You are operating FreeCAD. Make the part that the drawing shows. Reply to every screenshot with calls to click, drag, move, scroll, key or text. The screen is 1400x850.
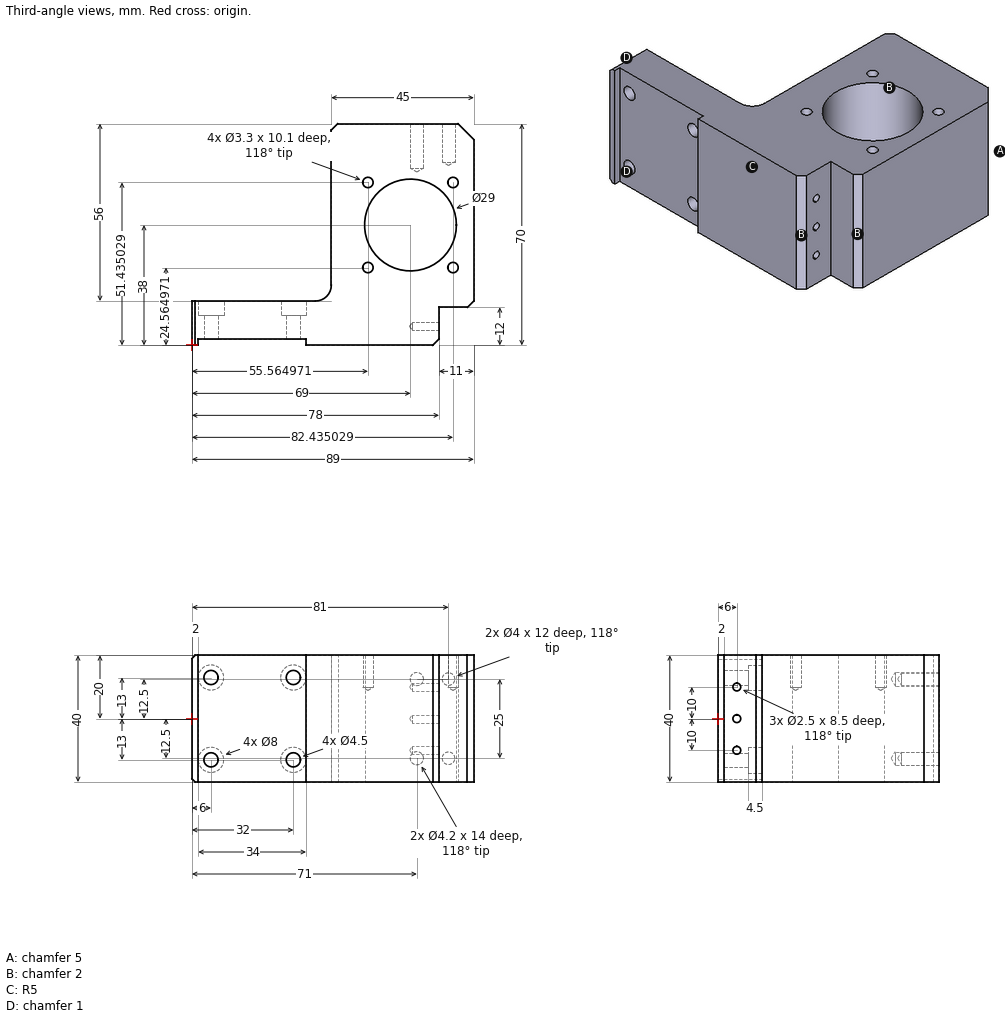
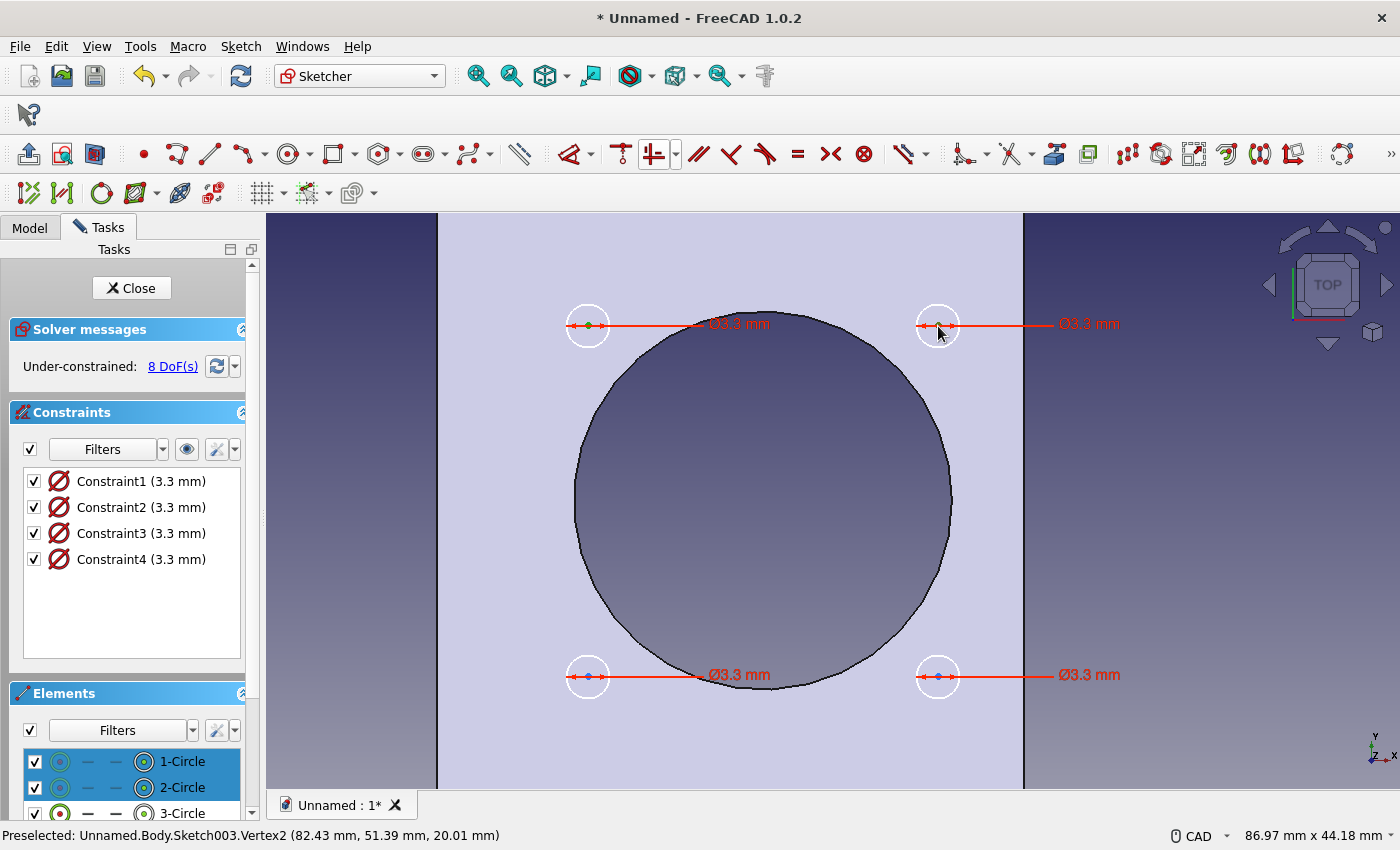
click(676, 154)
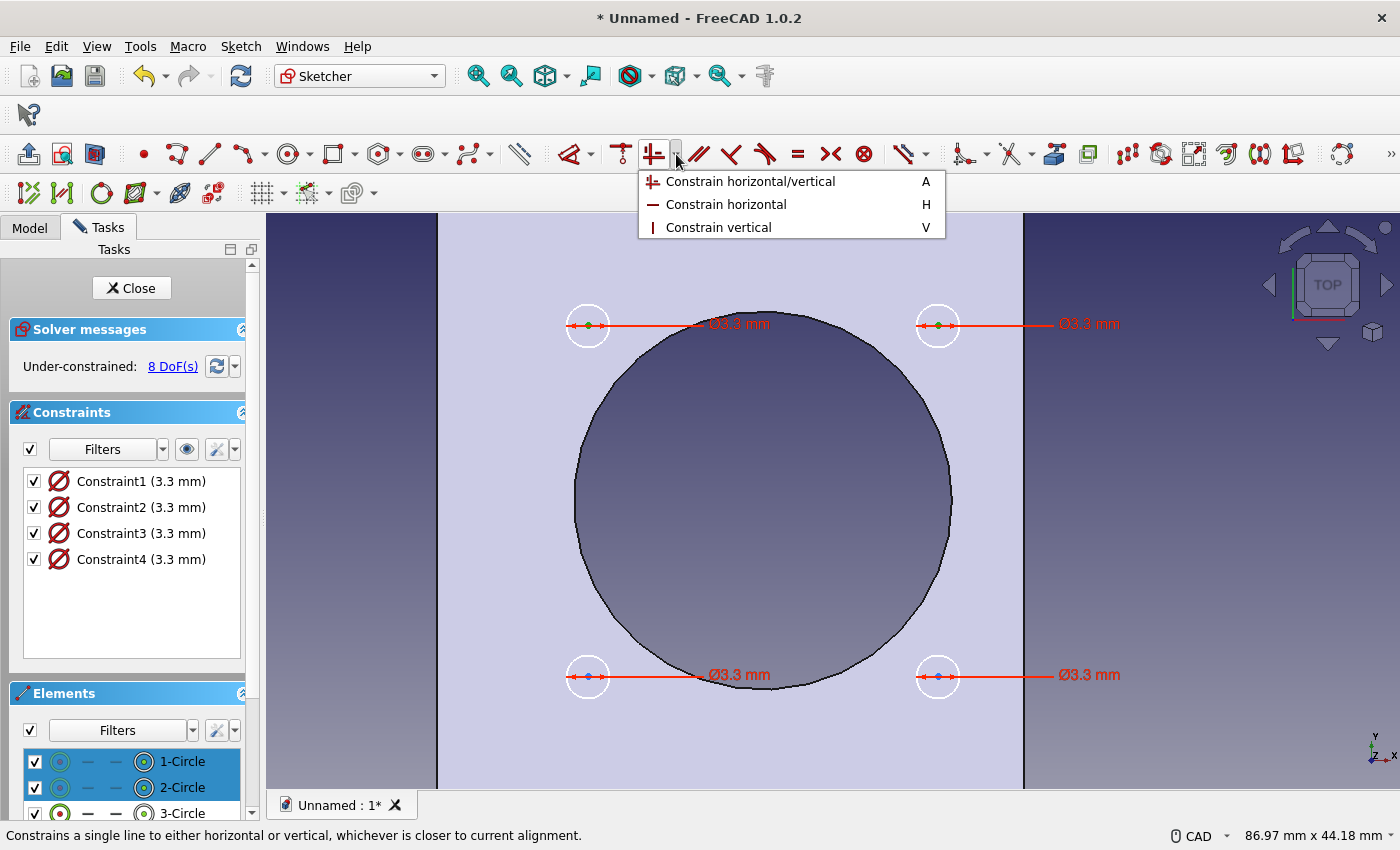
click(792, 204)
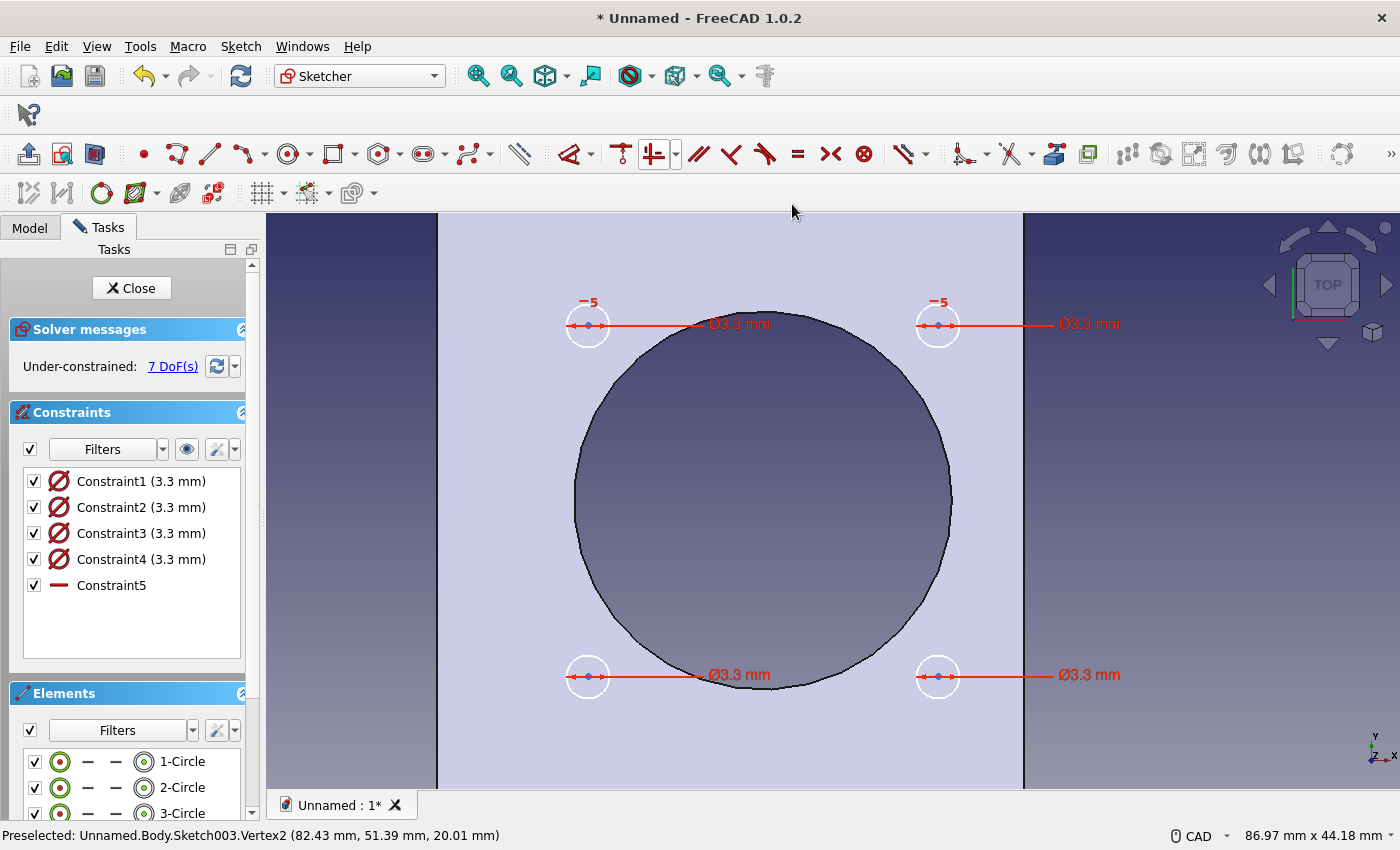
click(588, 326)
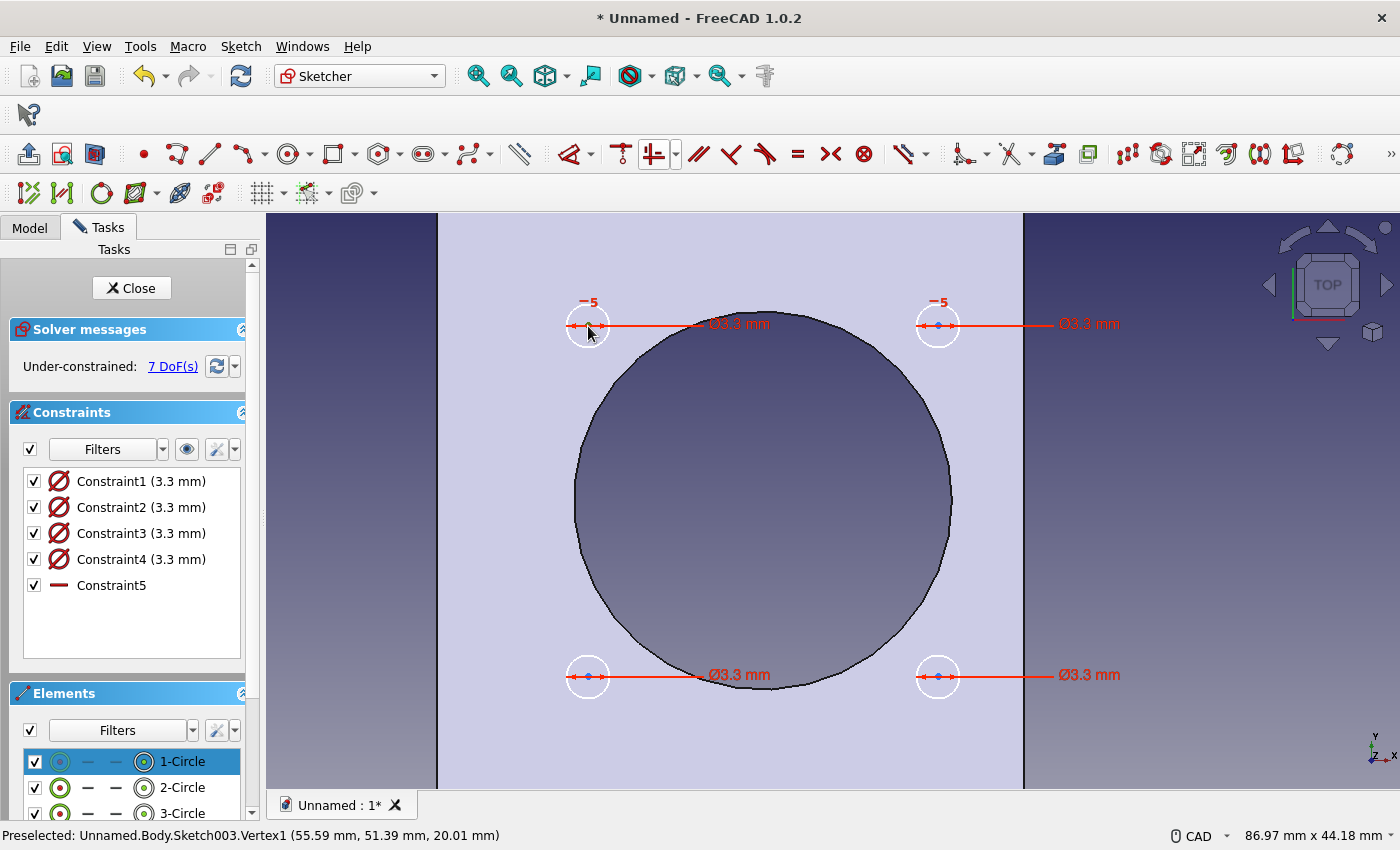
click(588, 677)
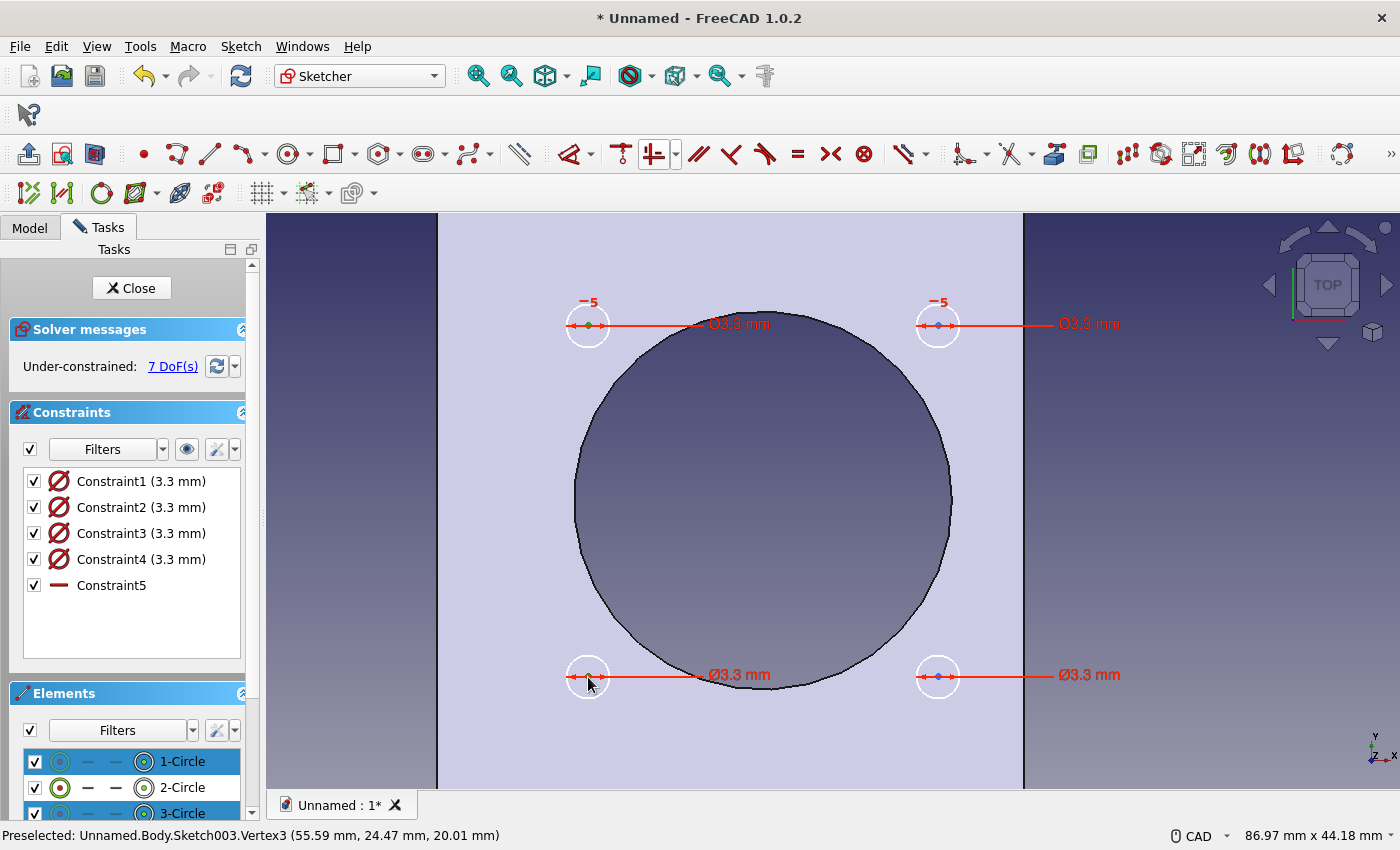
click(676, 154)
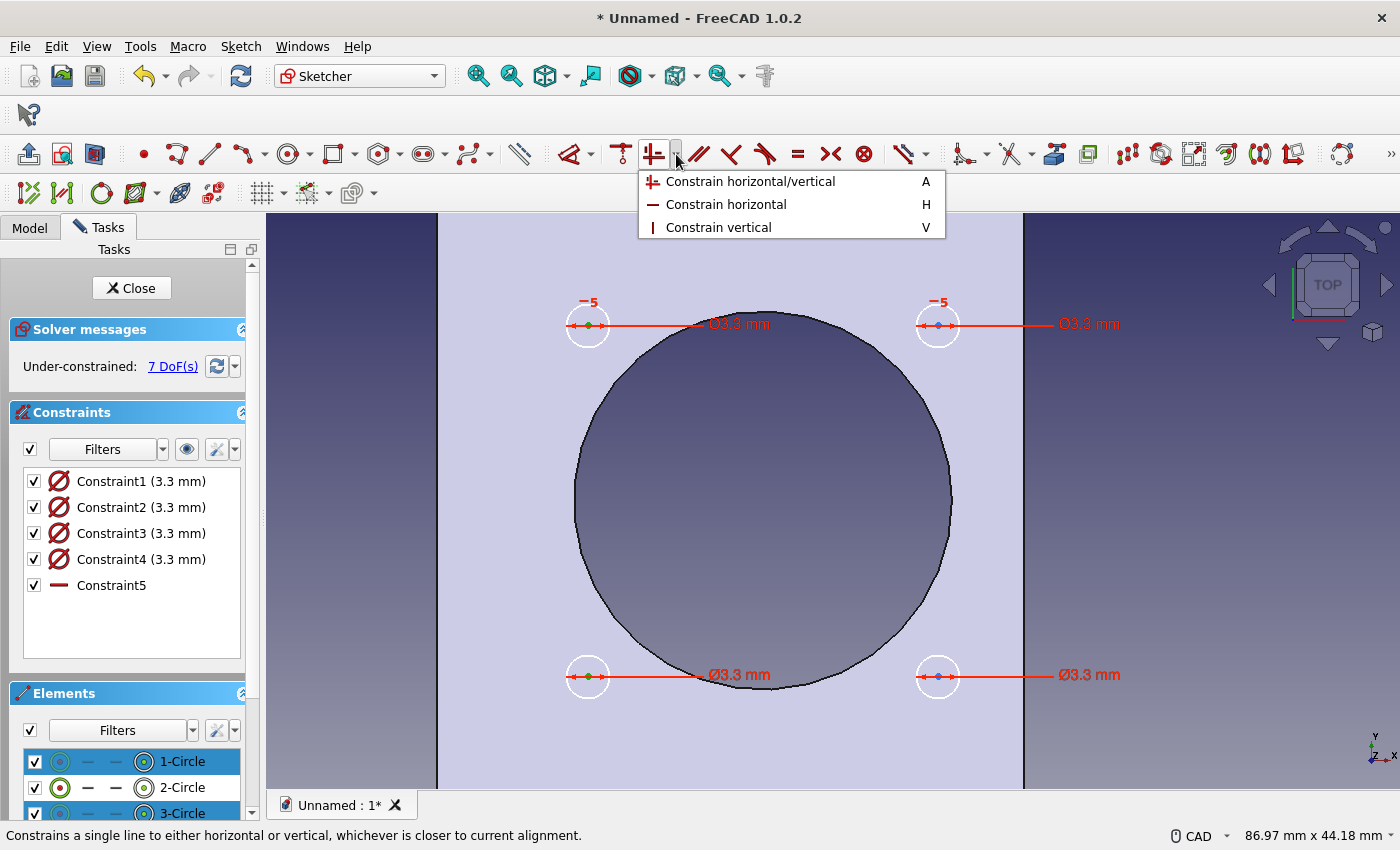
click(792, 228)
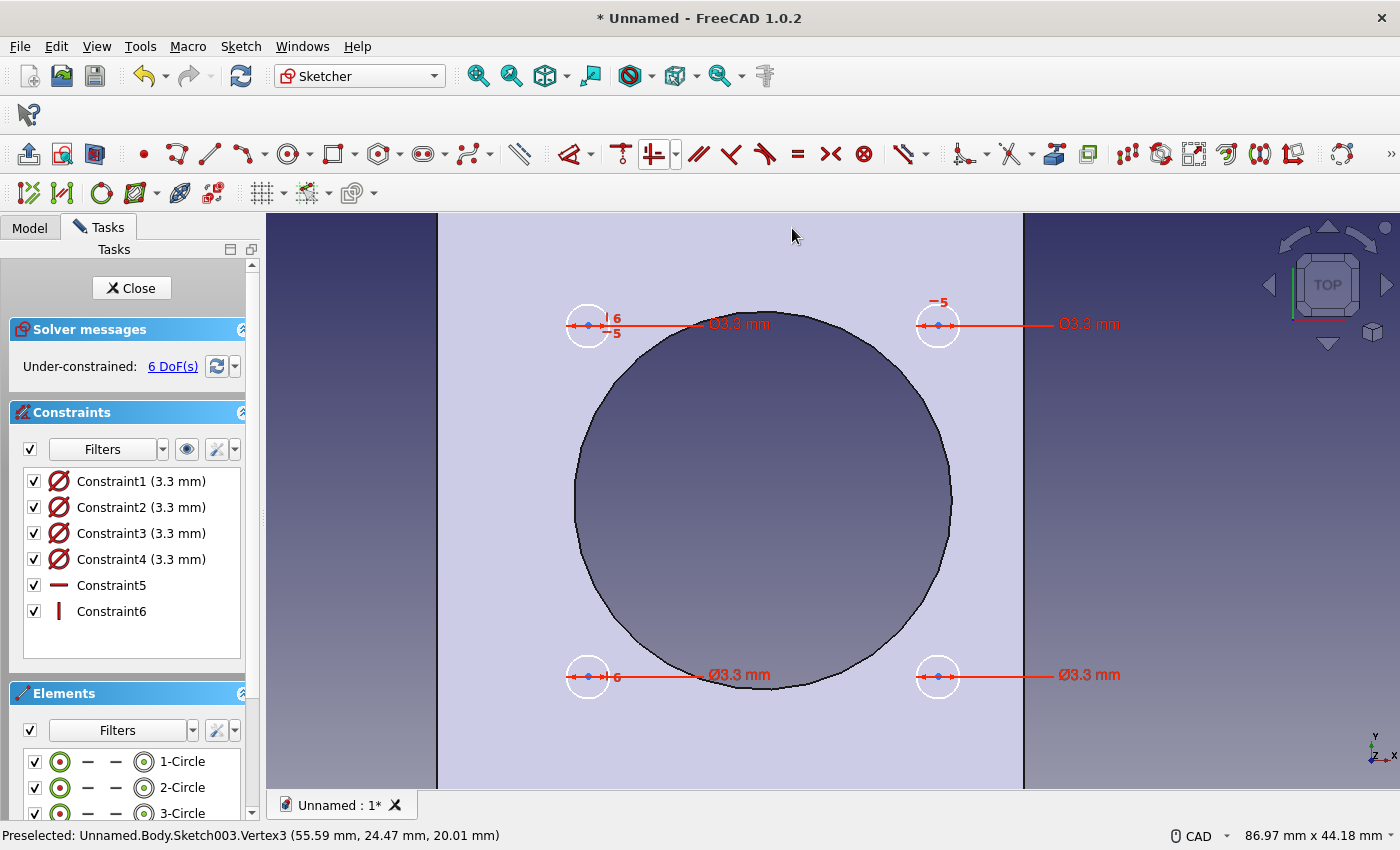
click(938, 326)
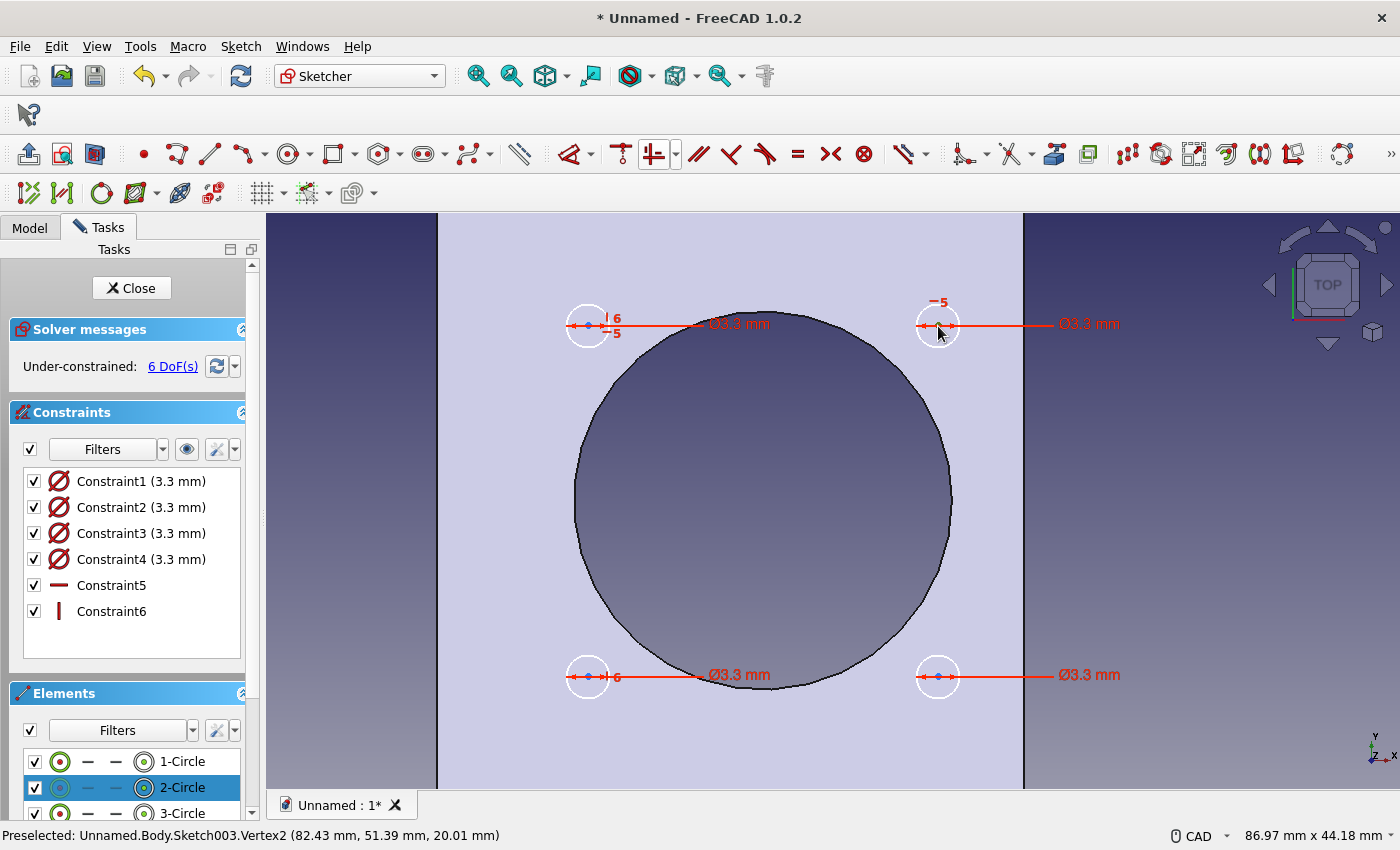
click(938, 677)